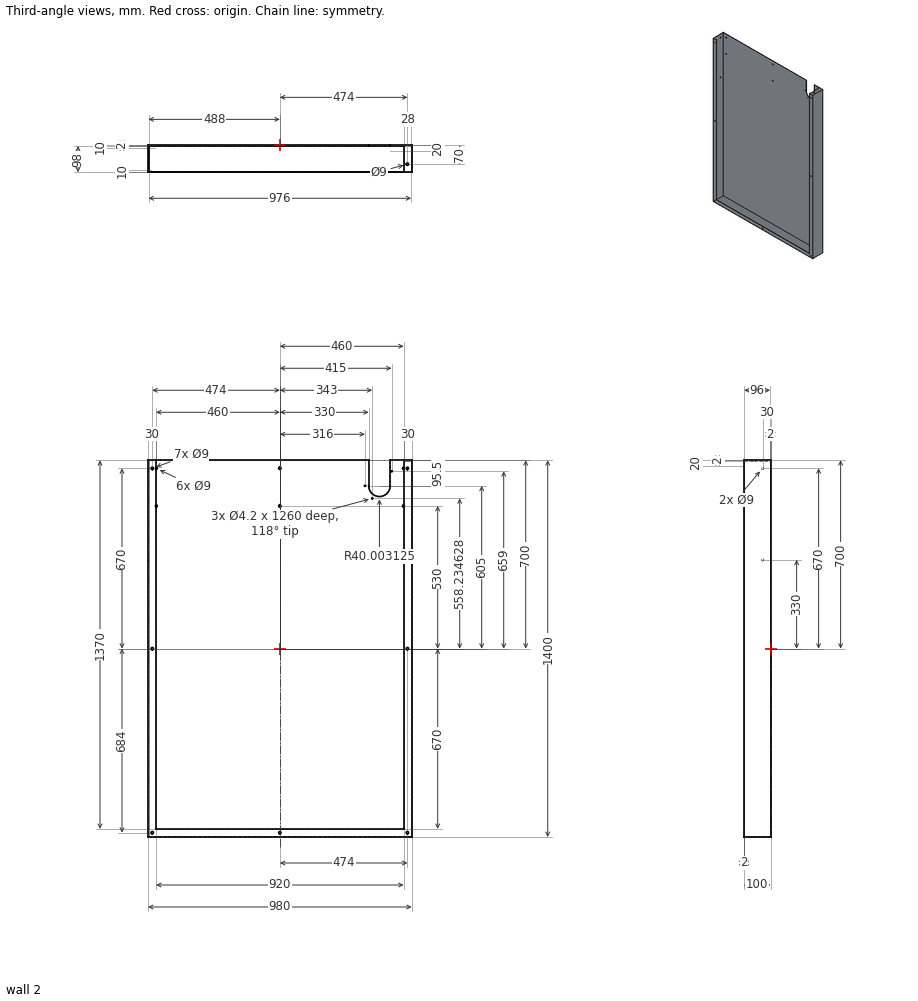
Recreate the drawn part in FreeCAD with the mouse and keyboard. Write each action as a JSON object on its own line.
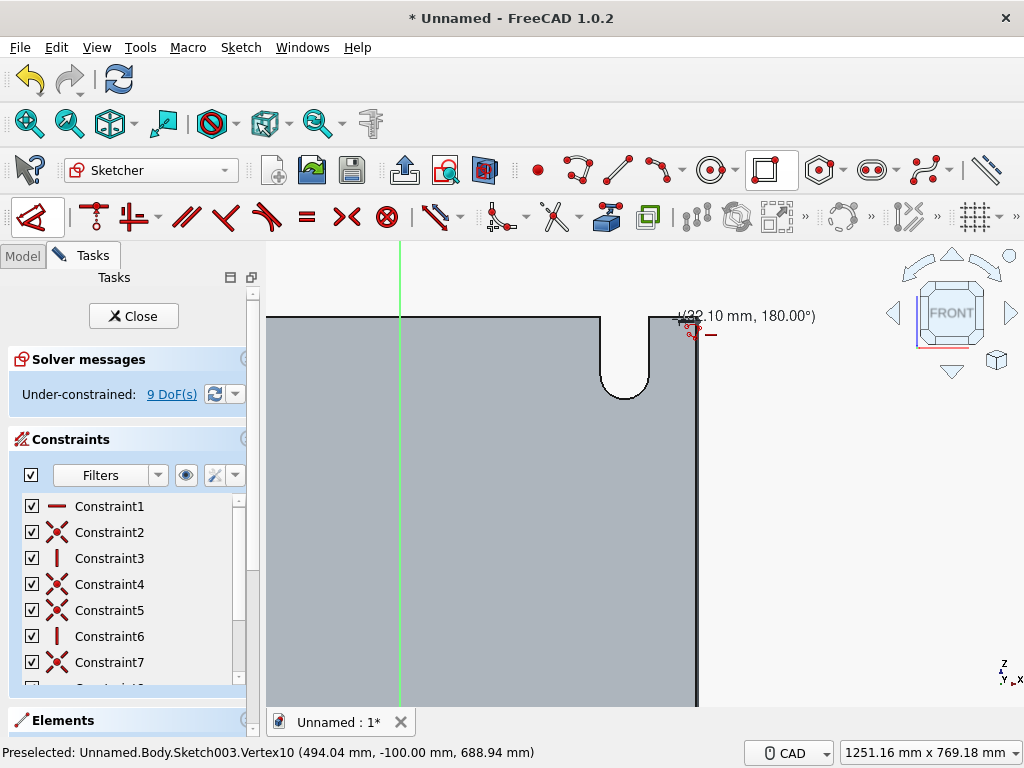
{"action": "left_click", "coordinate": [679, 319]}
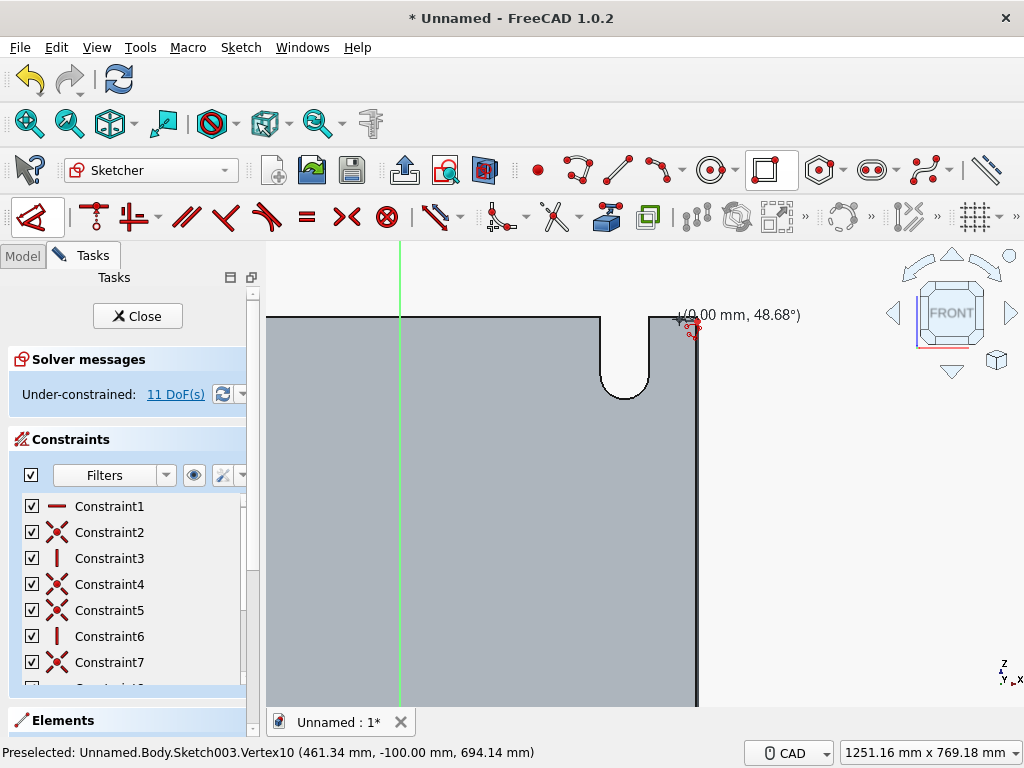
{"action": "scroll", "coordinate": [679, 318], "scroll_direction": "down", "scroll_amount": 5}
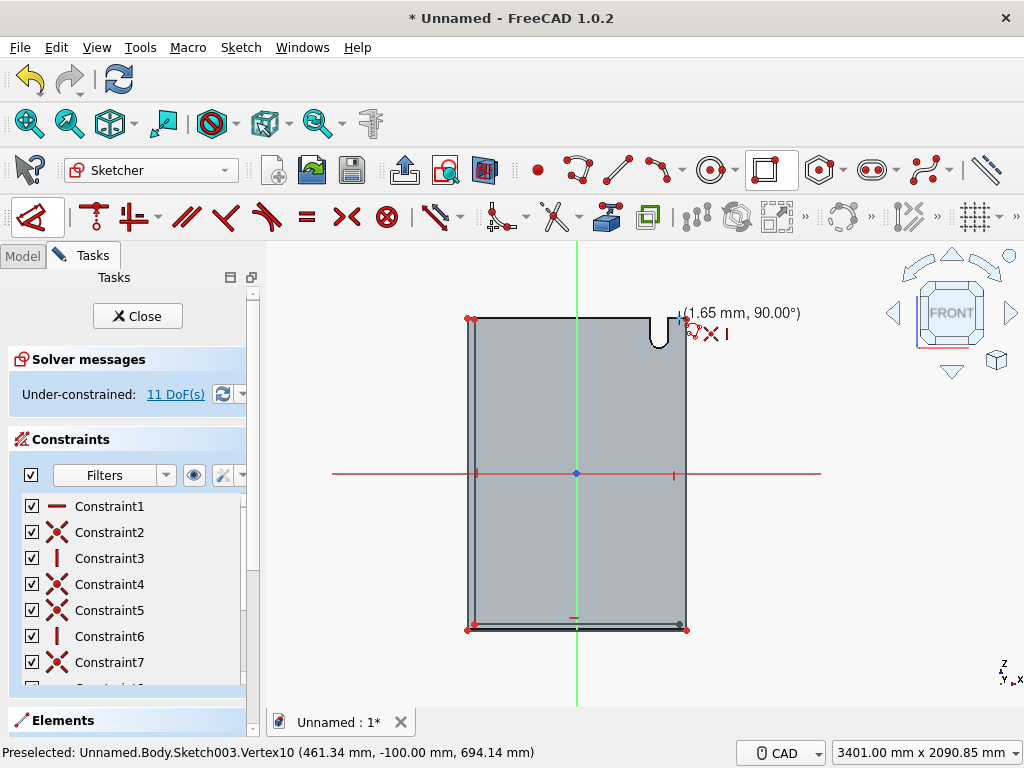
{"action": "scroll", "coordinate": [679, 623], "scroll_direction": "up", "scroll_amount": 5}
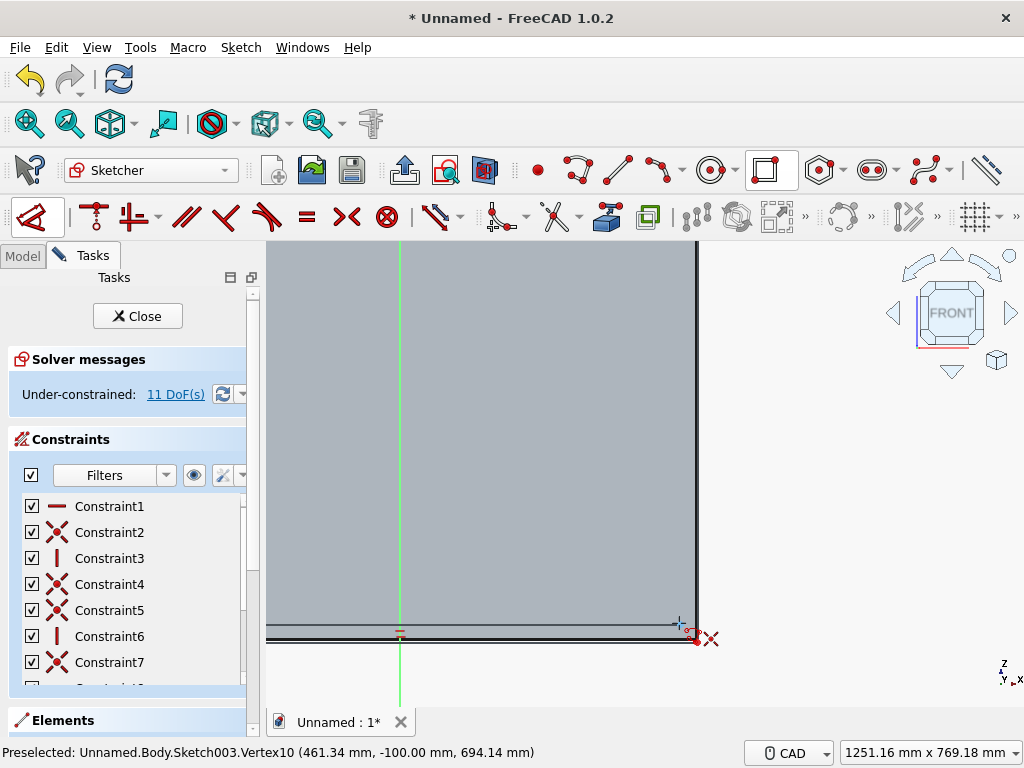
{"action": "left_click", "coordinate": [680, 625]}
{"action": "key", "text": "Escape"}
{"action": "key", "text": "Escape"}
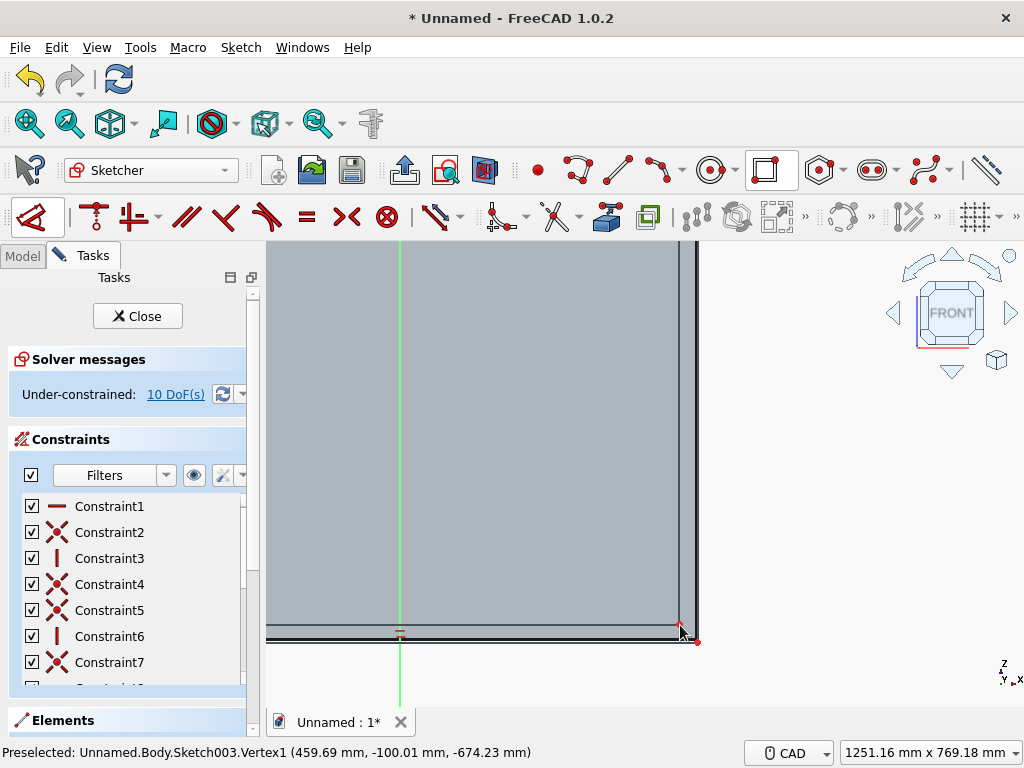
{"action": "scroll", "coordinate": [679, 624], "scroll_direction": "down", "scroll_amount": 5}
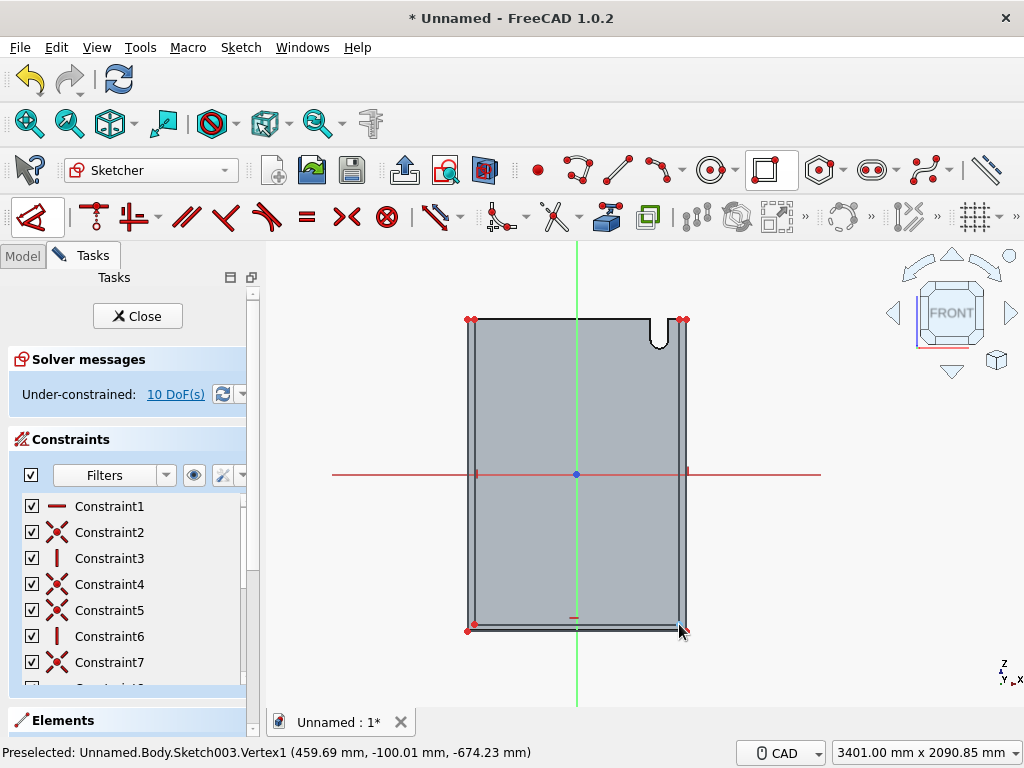
{"action": "scroll", "coordinate": [471, 320], "scroll_direction": "up", "scroll_amount": 7}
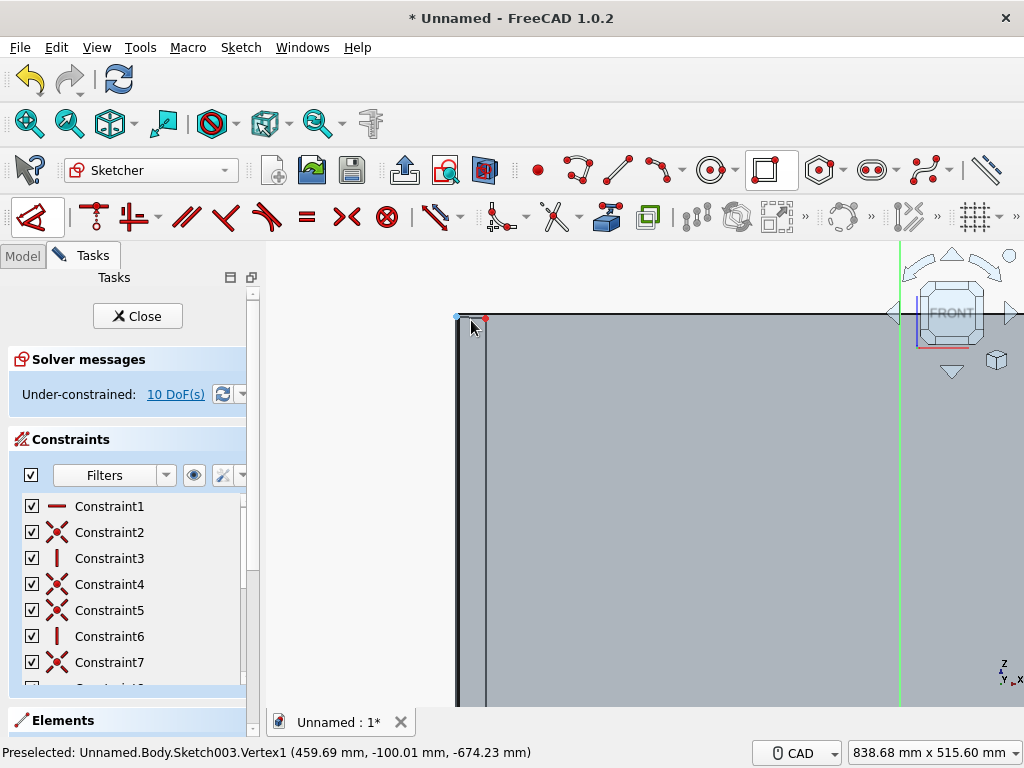
{"action": "left_click", "coordinate": [471, 318]}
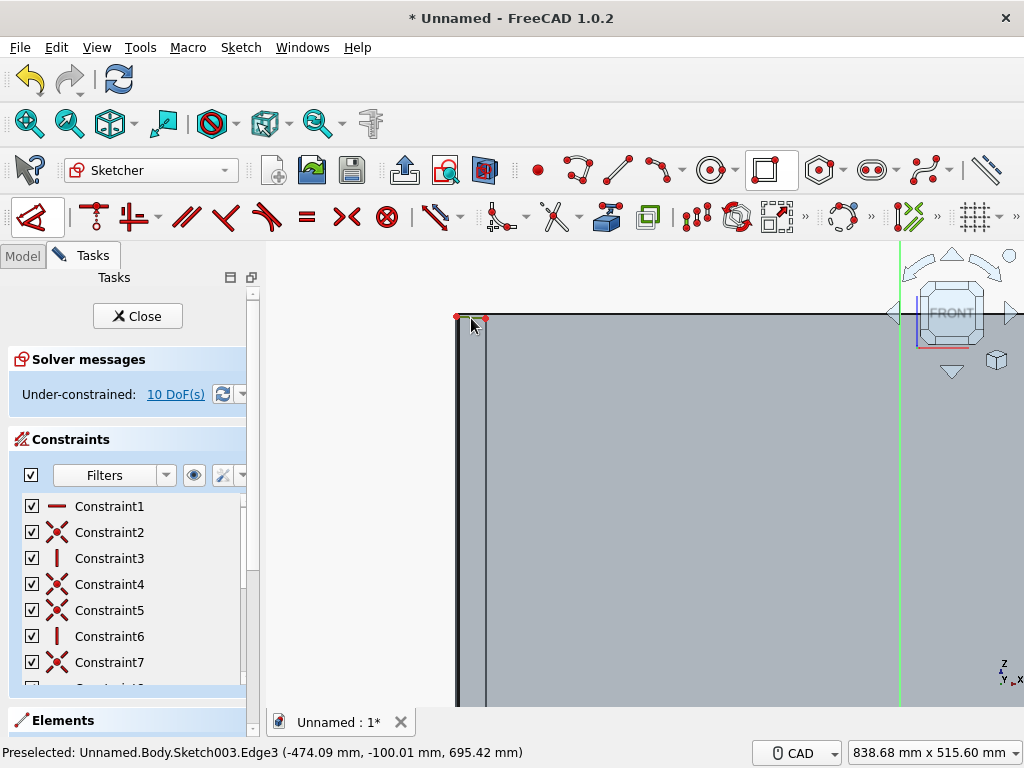
{"action": "key", "text": "h"}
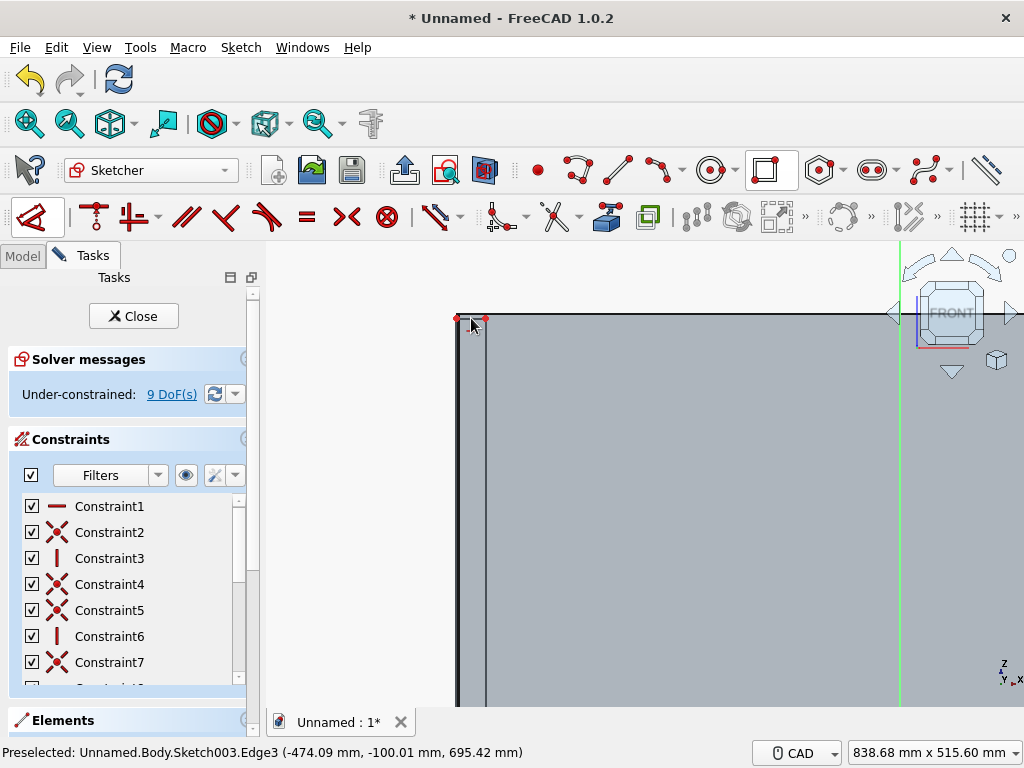
{"action": "scroll", "coordinate": [471, 319], "scroll_direction": "down", "scroll_amount": 7}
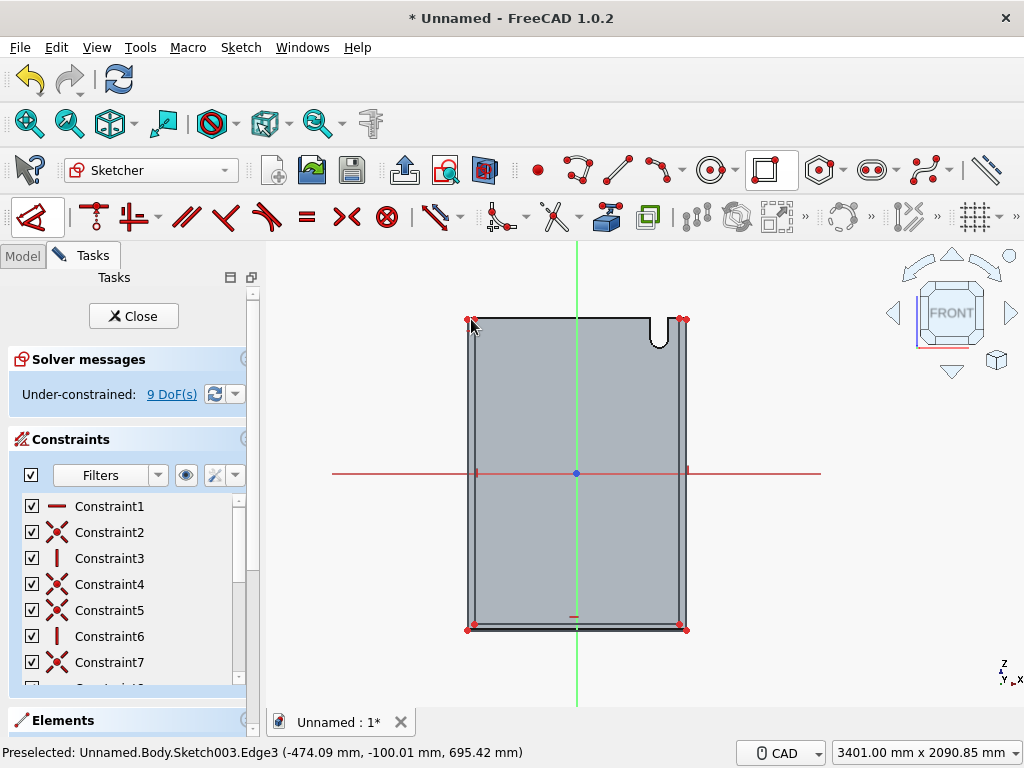
{"action": "scroll", "coordinate": [683, 319], "scroll_direction": "up", "scroll_amount": 9}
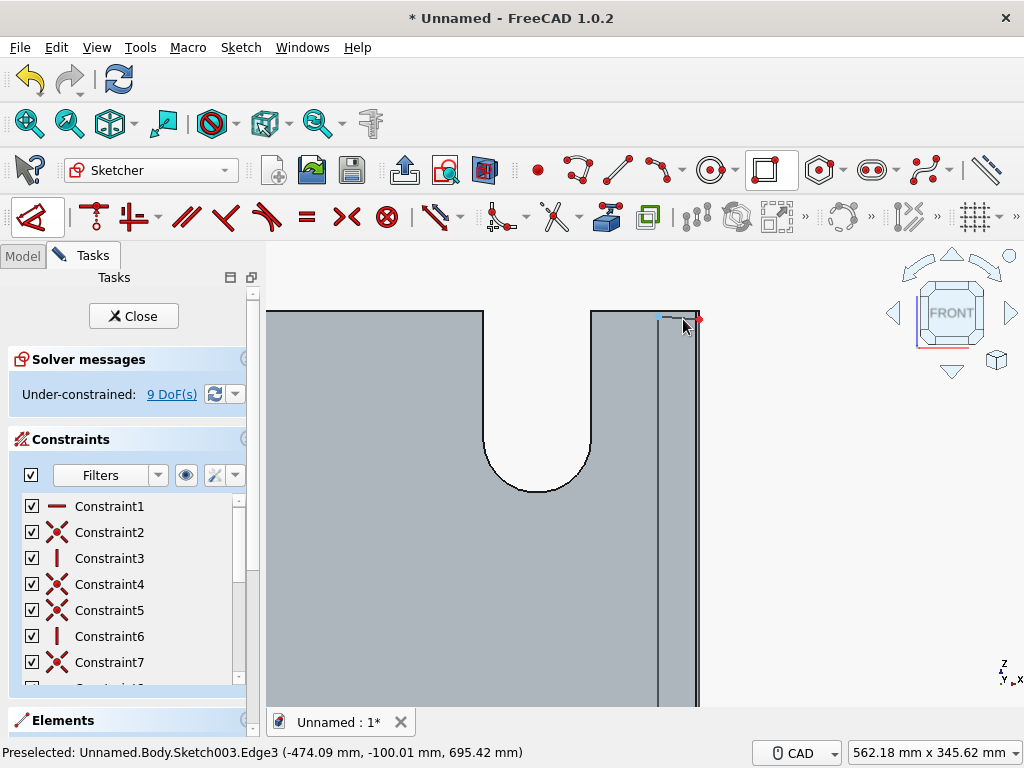
{"action": "left_click", "coordinate": [683, 318]}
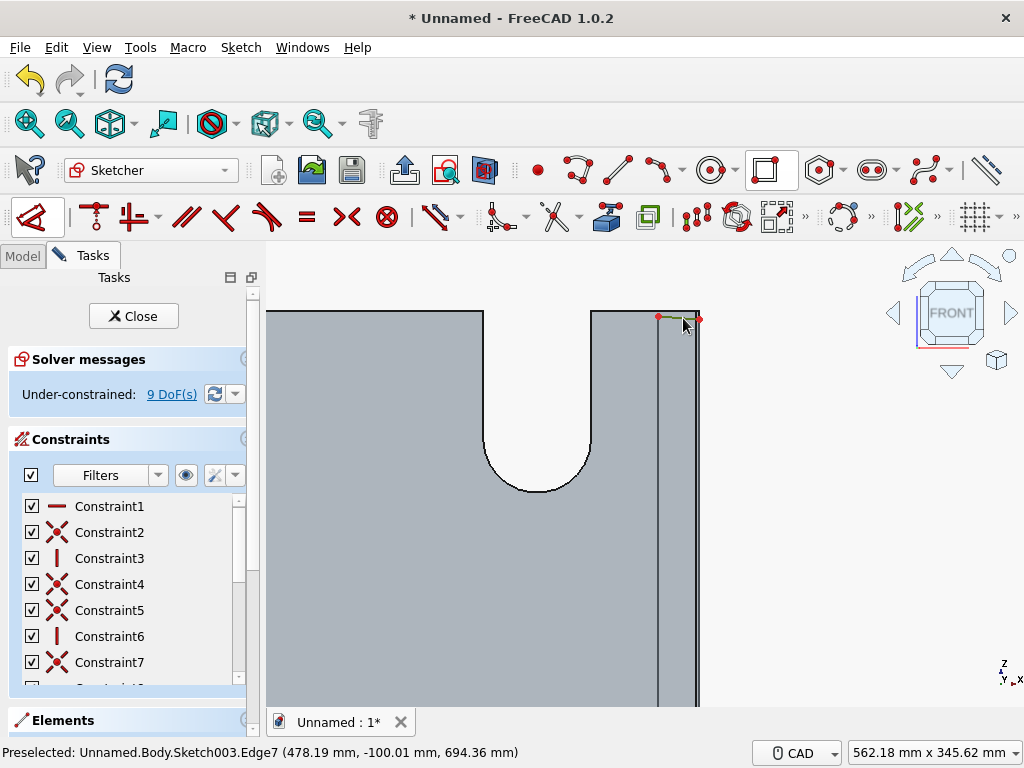
{"action": "left_click", "coordinate": [160, 218]}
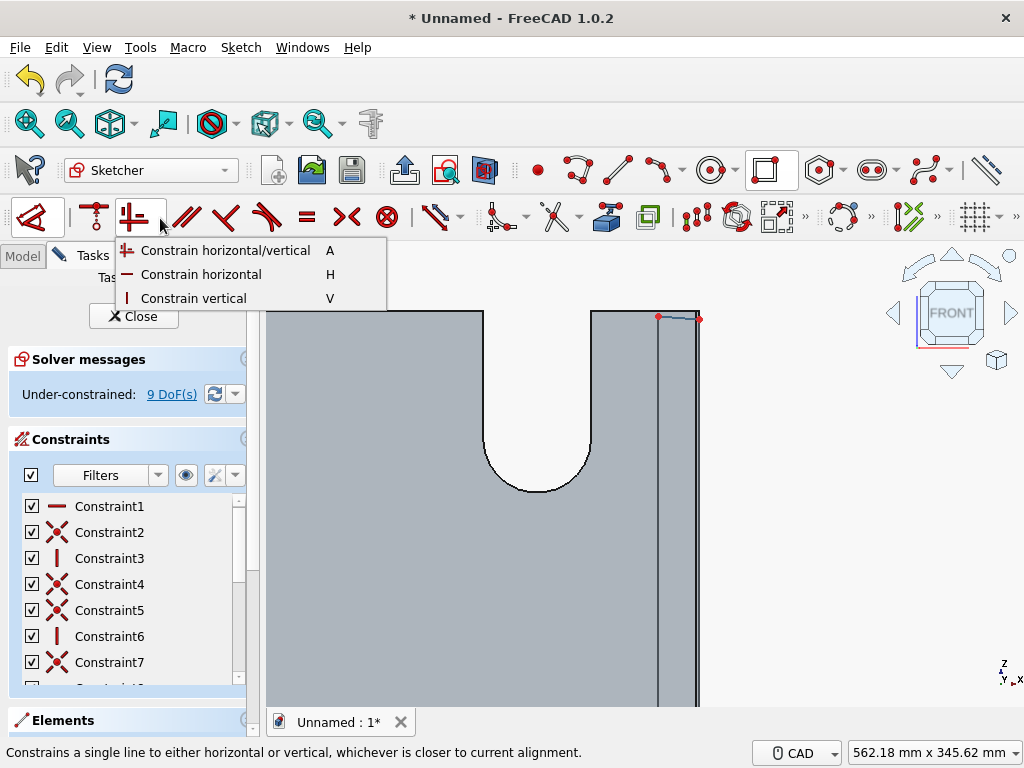
{"action": "left_click", "coordinate": [251, 274]}